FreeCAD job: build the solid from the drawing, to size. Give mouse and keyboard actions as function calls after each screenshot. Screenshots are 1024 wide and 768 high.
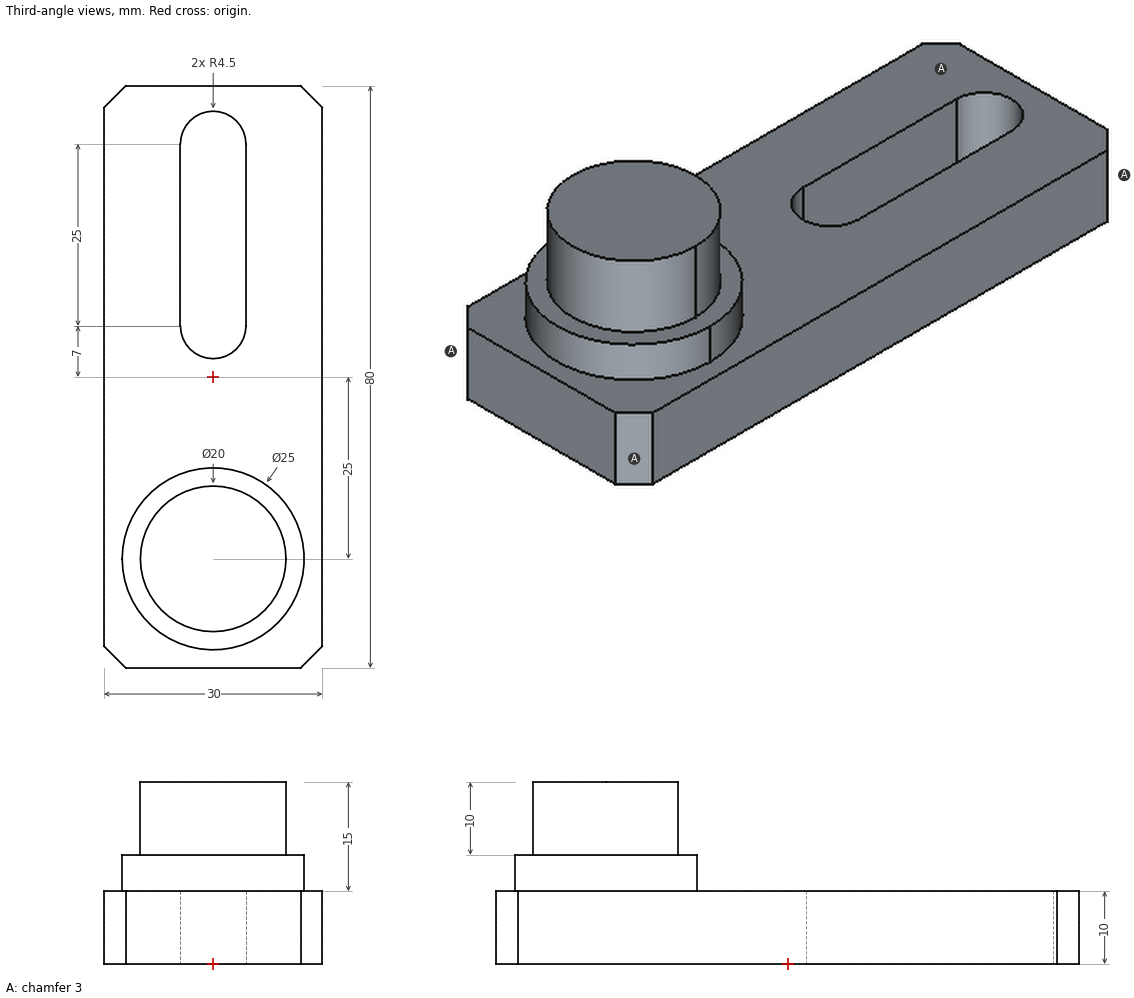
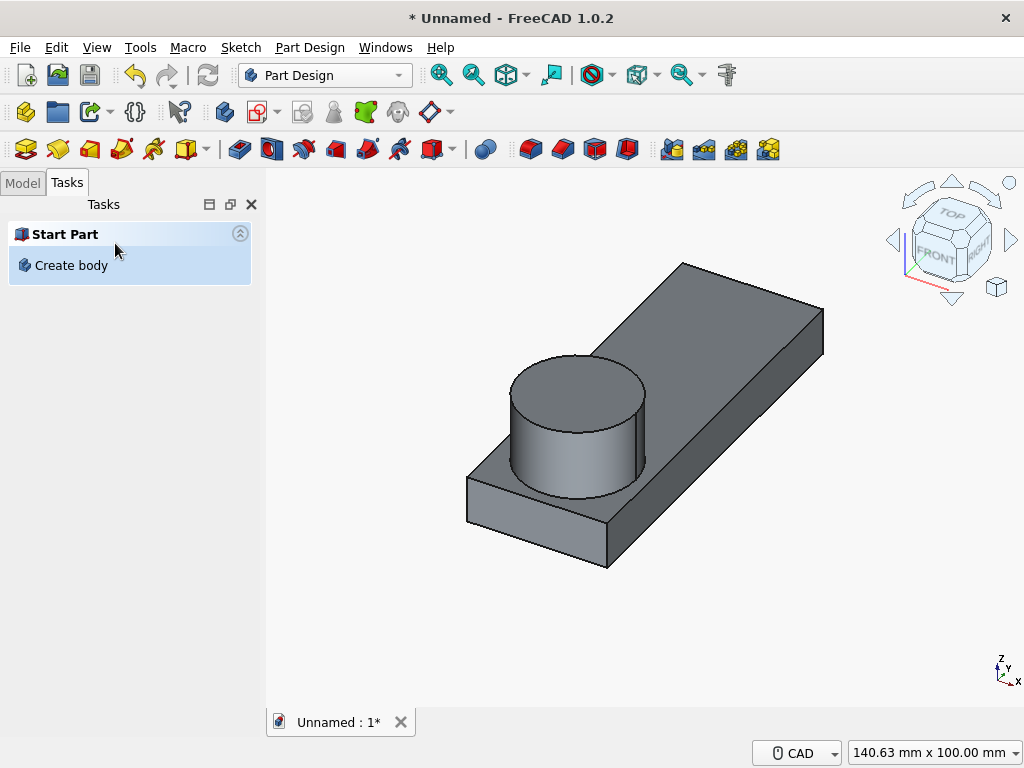
click(23, 182)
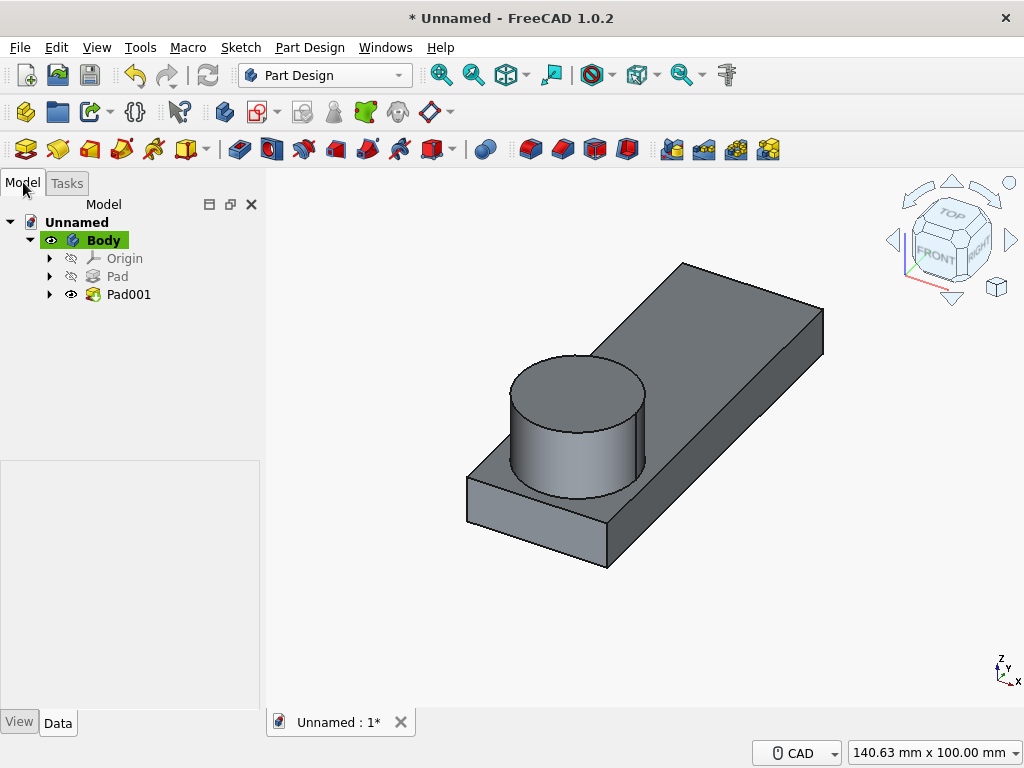
click(50, 258)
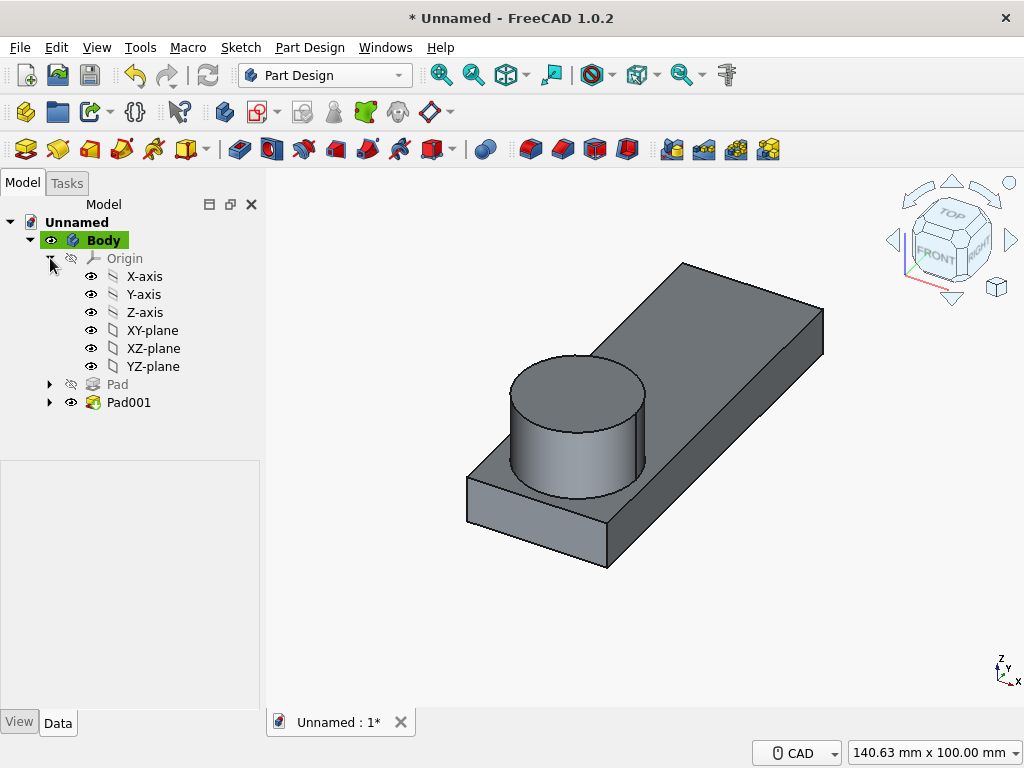
click(136, 330)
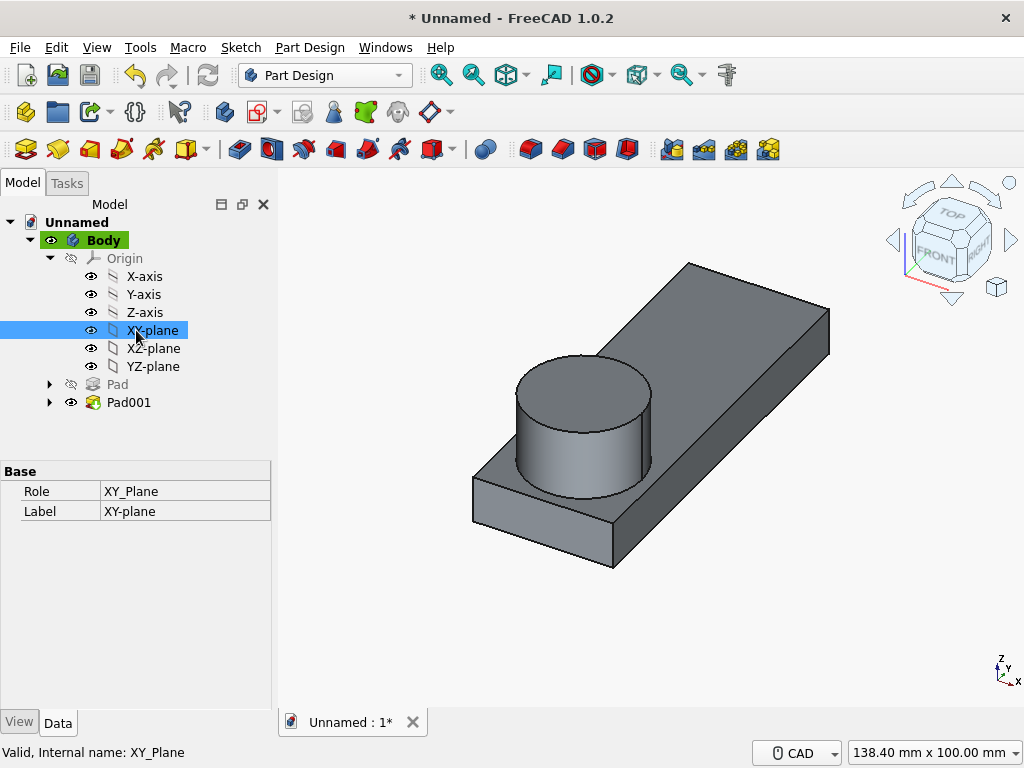
click(430, 112)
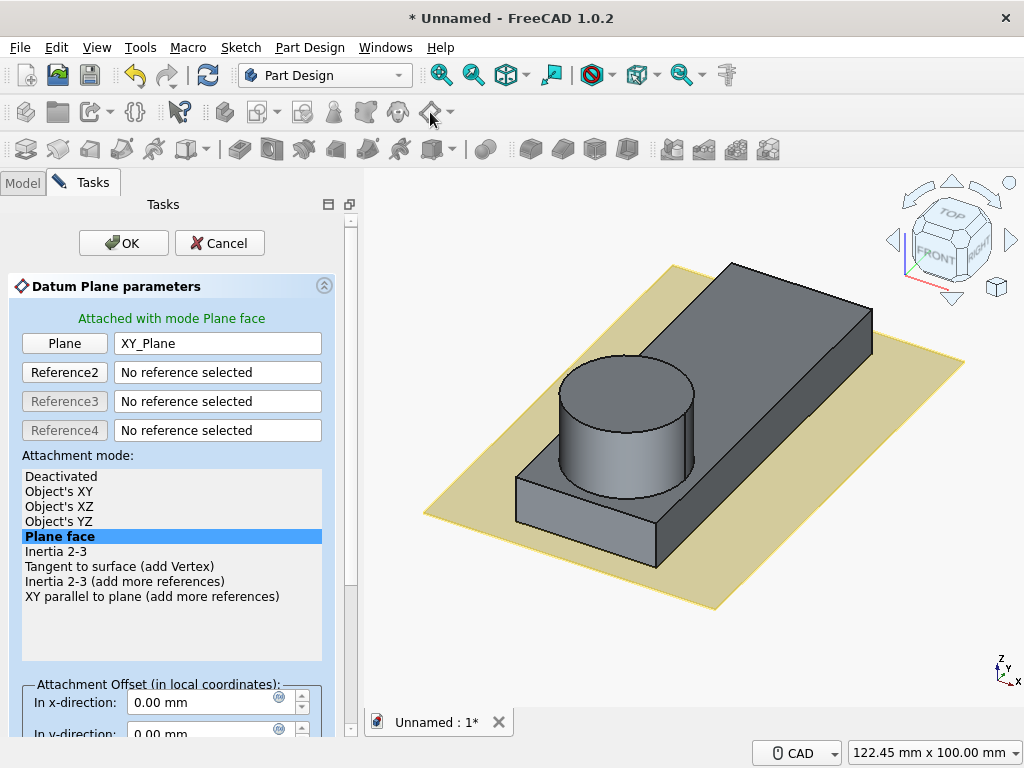
scroll(351, 475, down, 2)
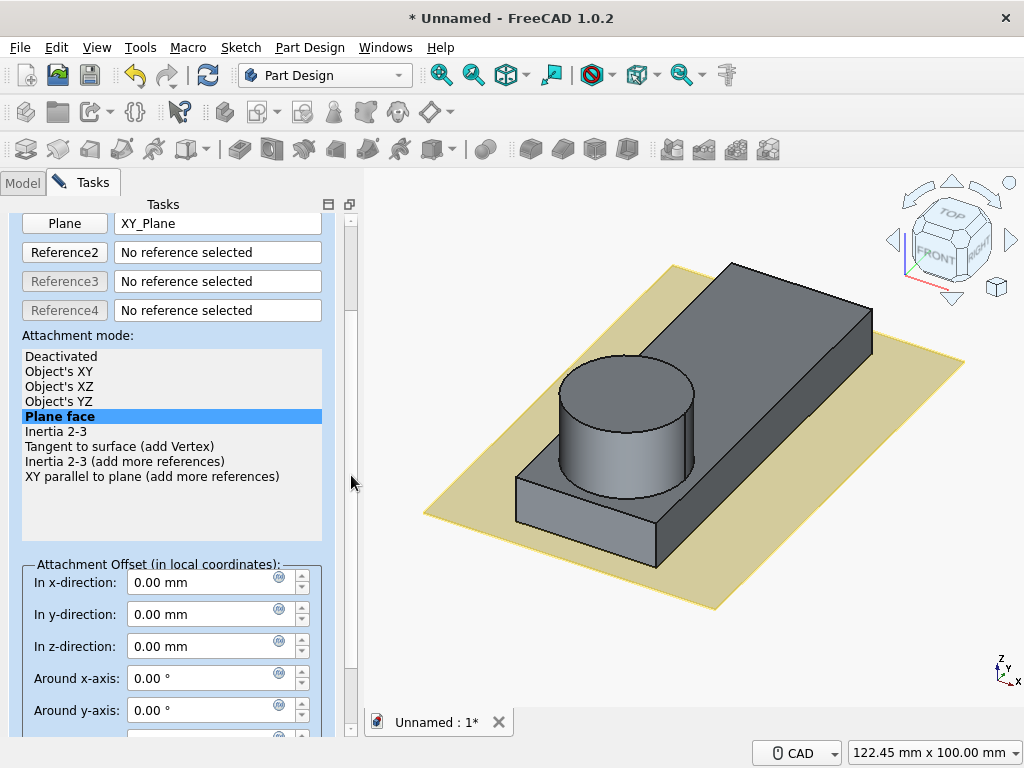
triple_click(210, 646)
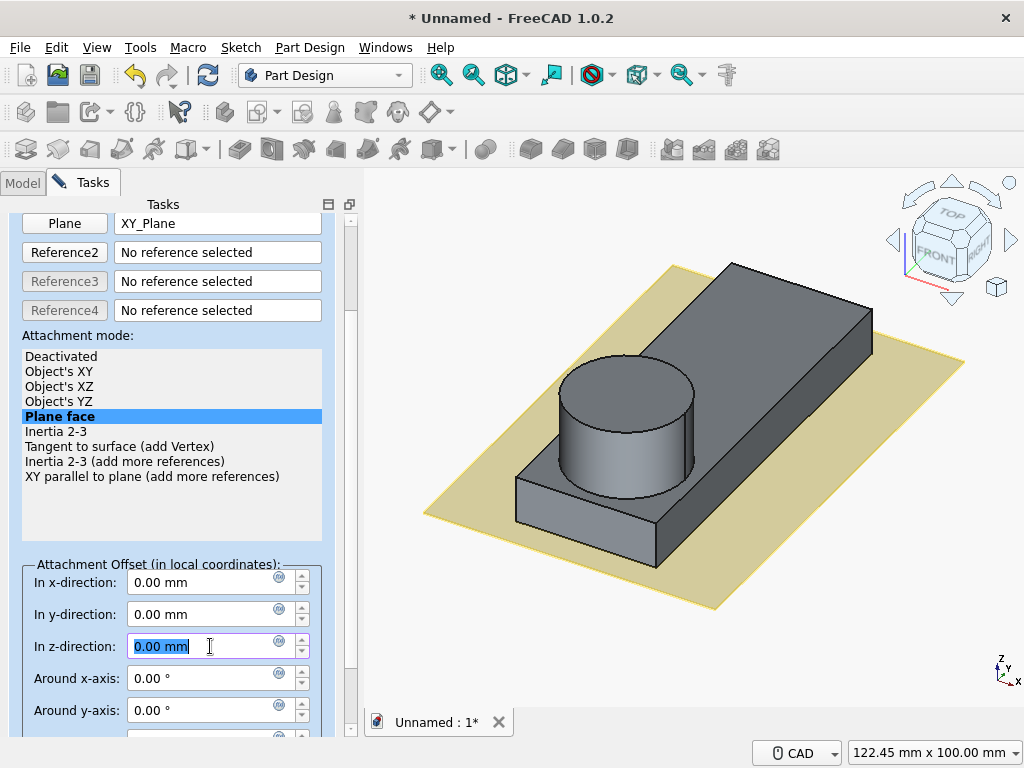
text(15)
key(Tab)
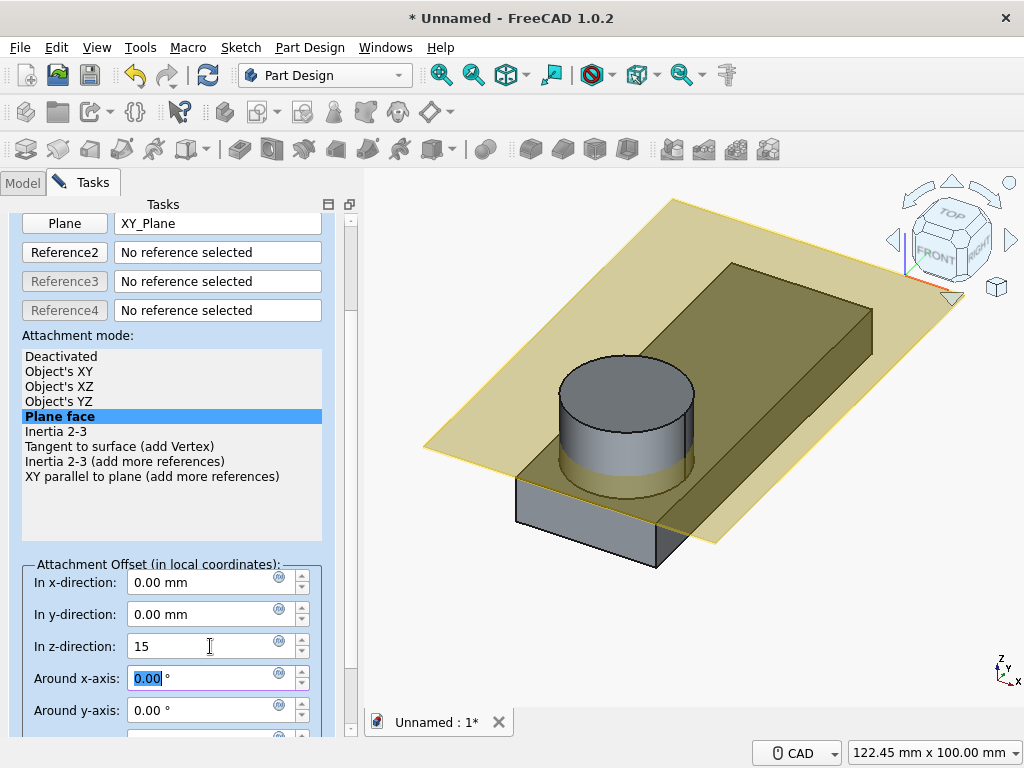
scroll(351, 475, up, 3)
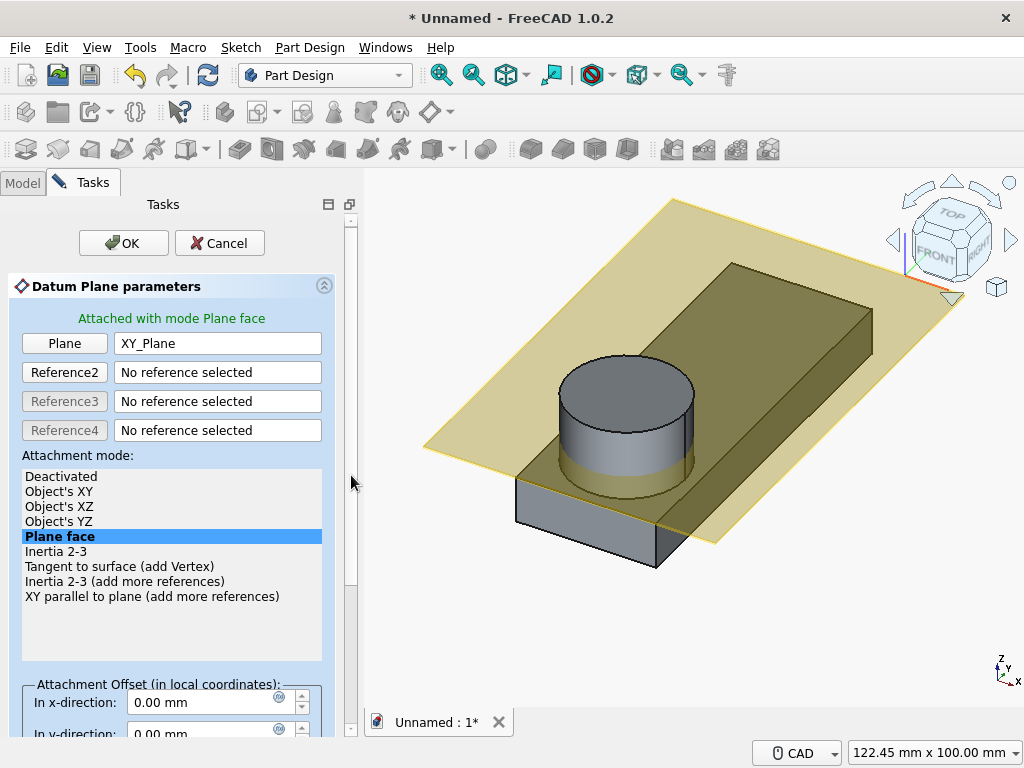
click(124, 243)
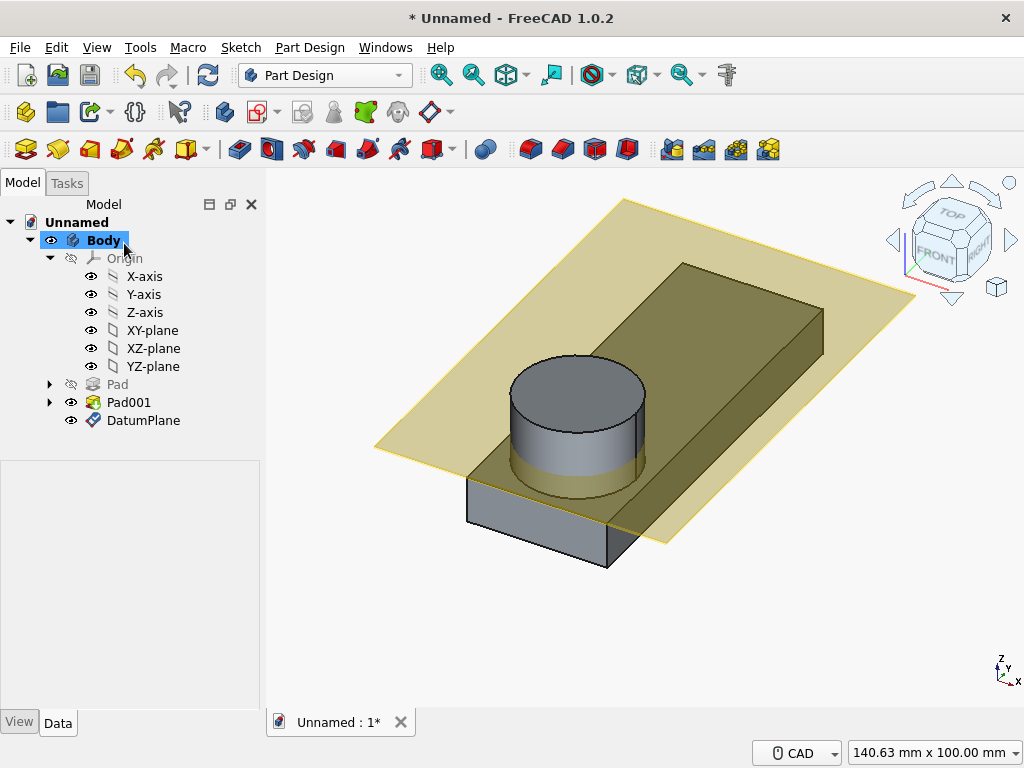
click(116, 420)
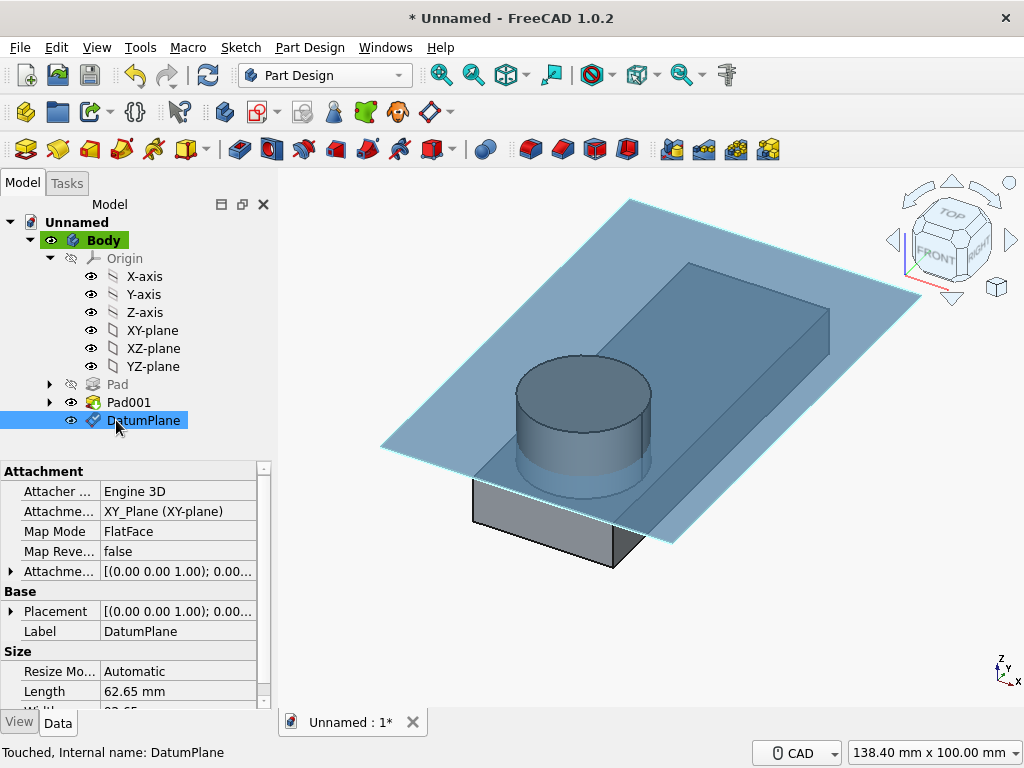
click(258, 112)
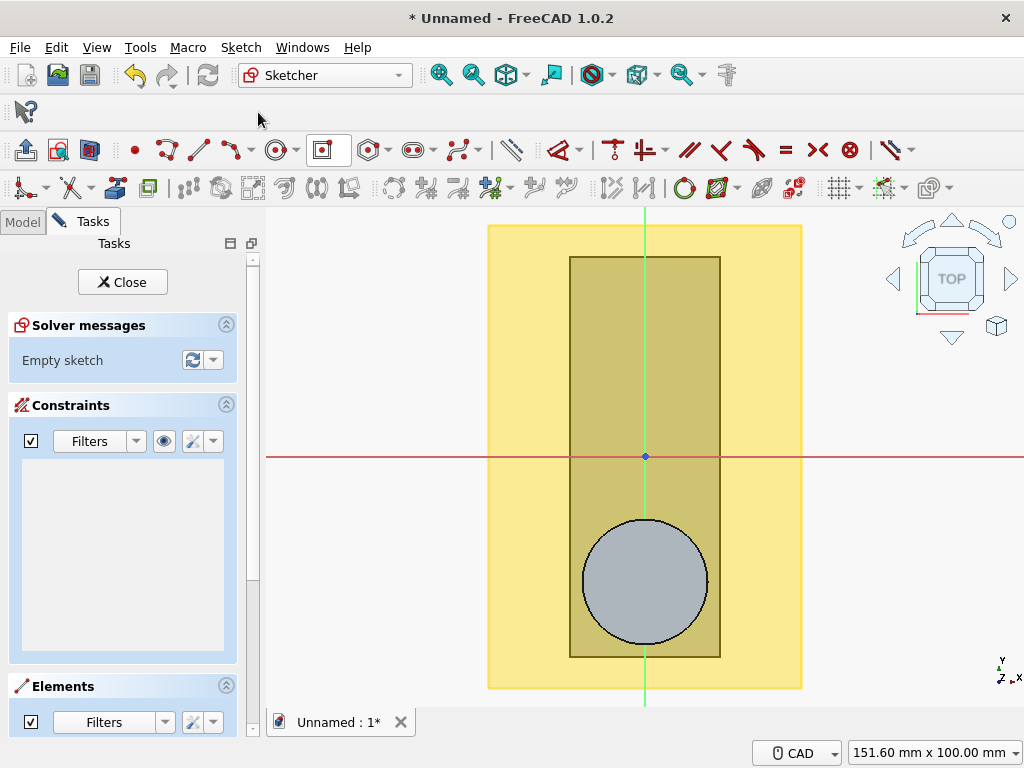
click(90, 150)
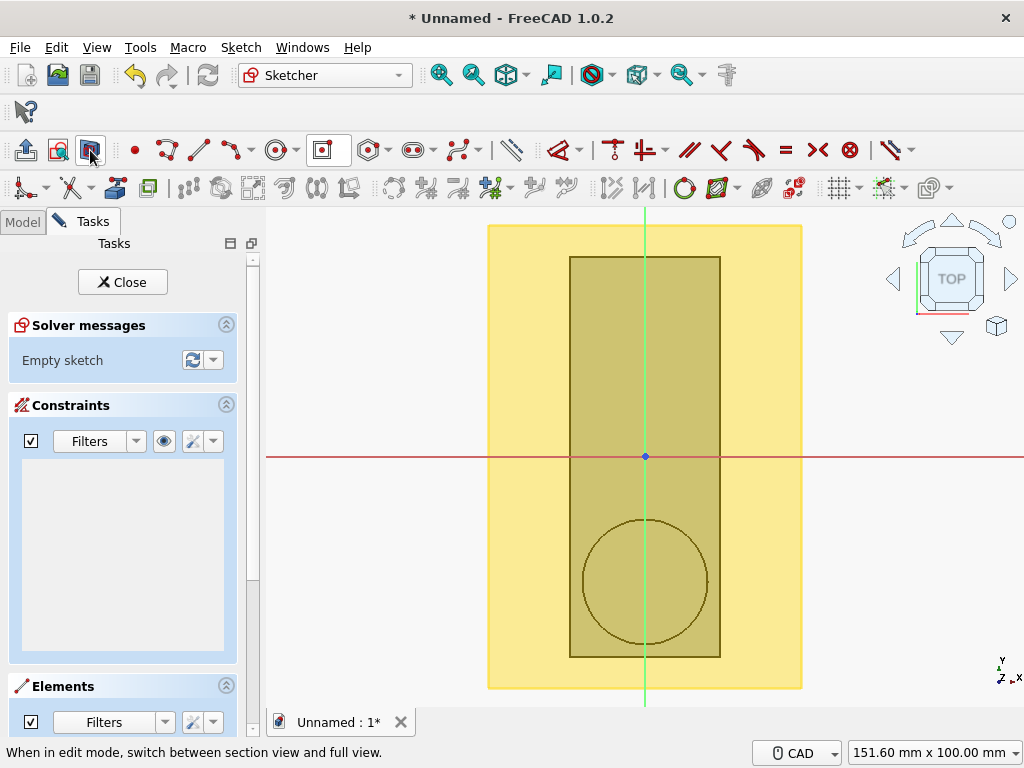
scroll(728, 665, up, 3)